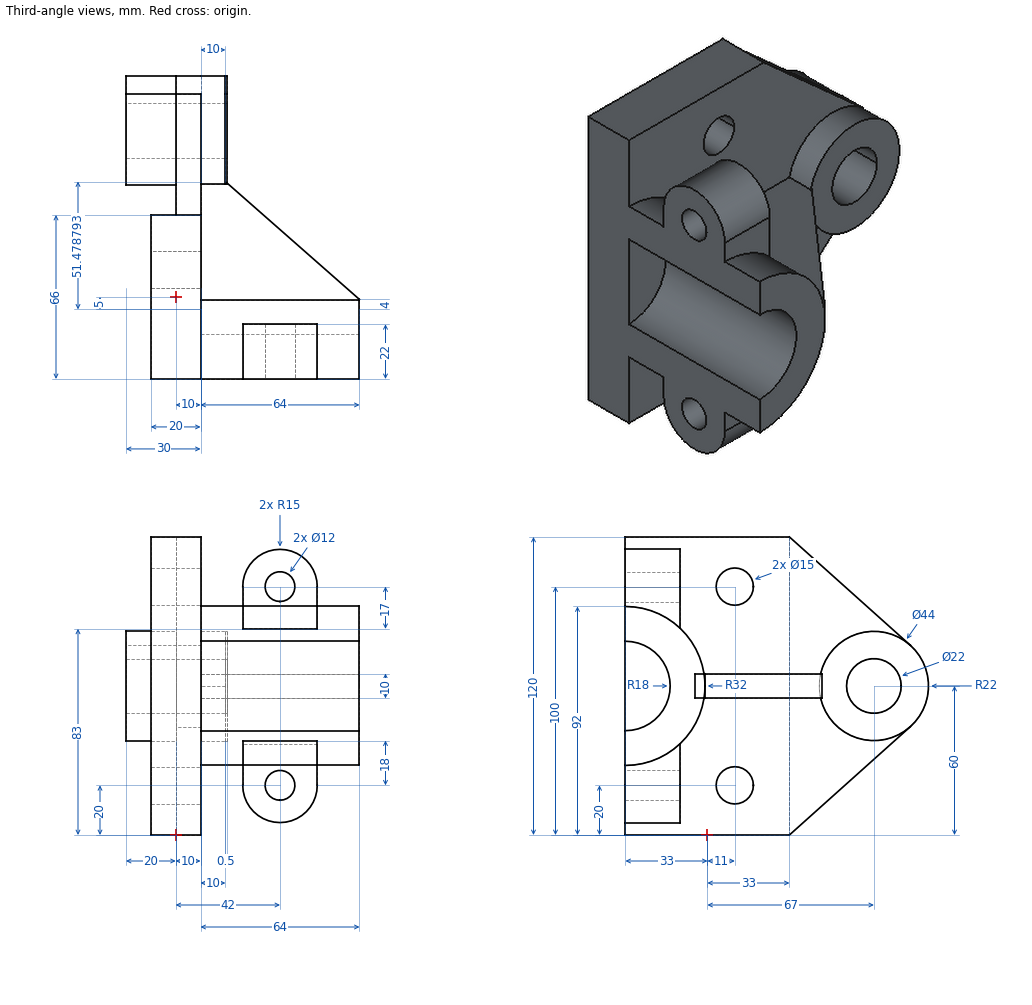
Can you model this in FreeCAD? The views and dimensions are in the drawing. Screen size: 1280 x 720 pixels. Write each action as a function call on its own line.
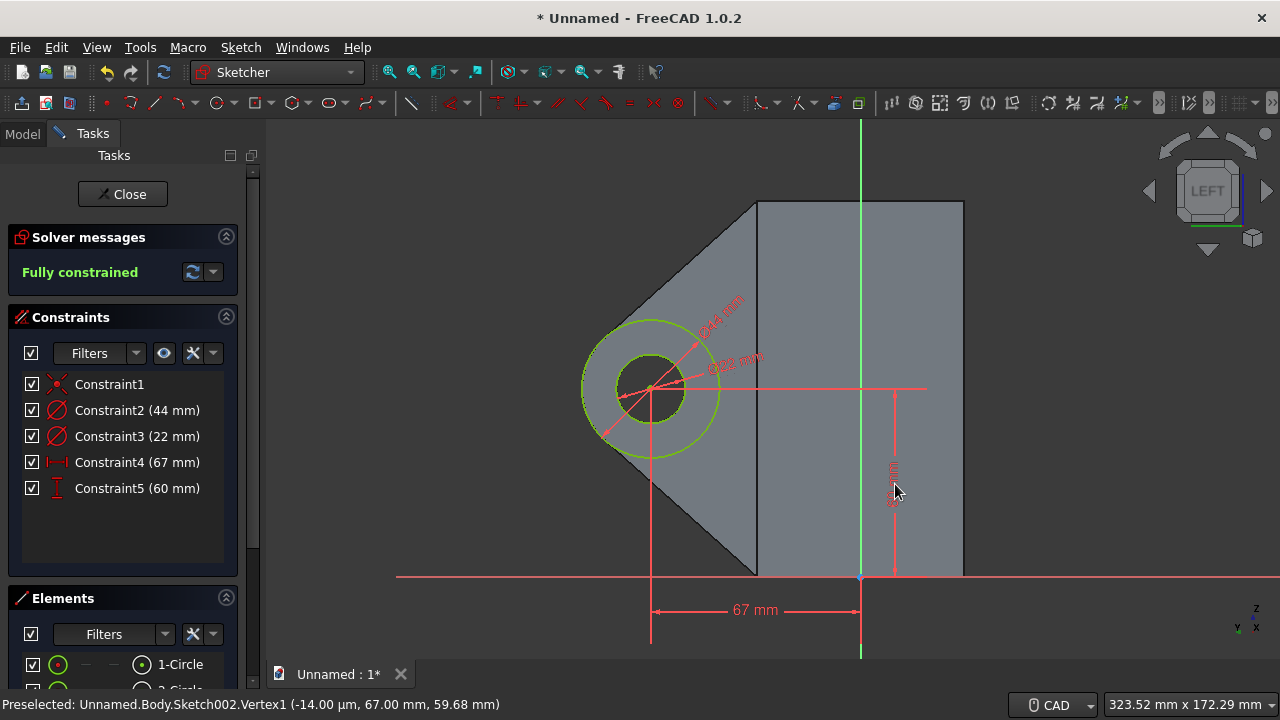
click(123, 194)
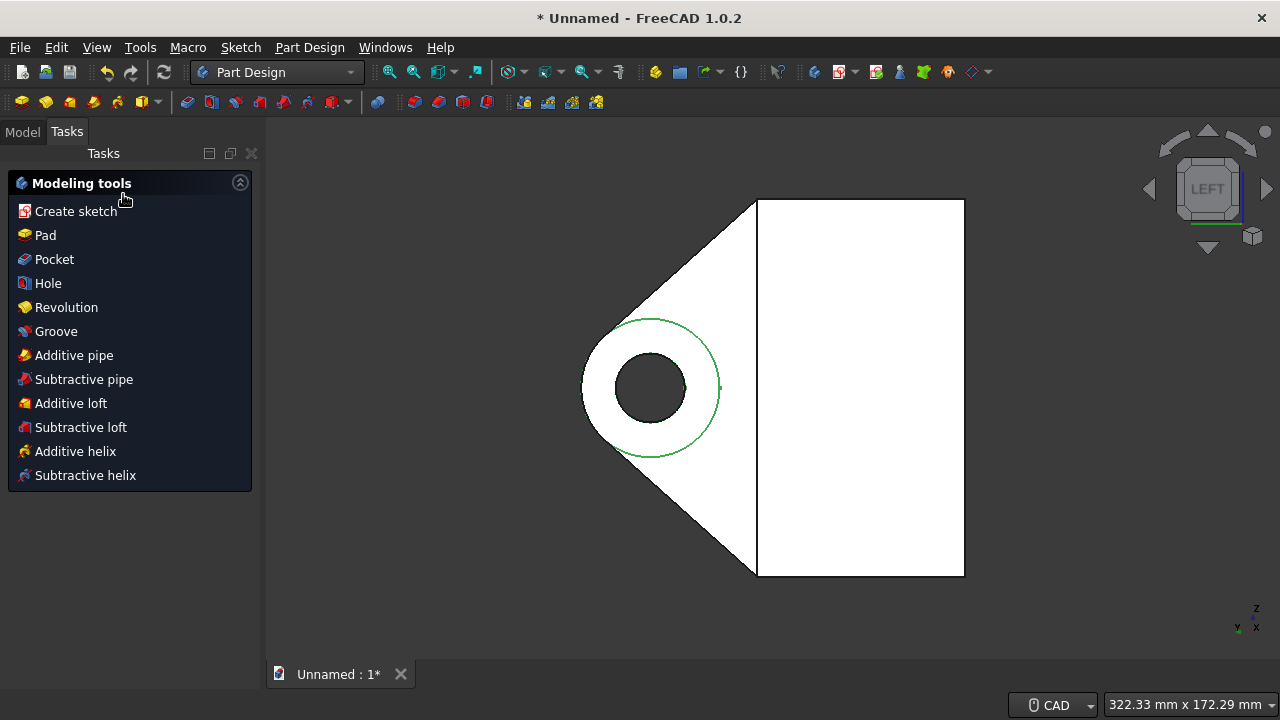
click(22, 102)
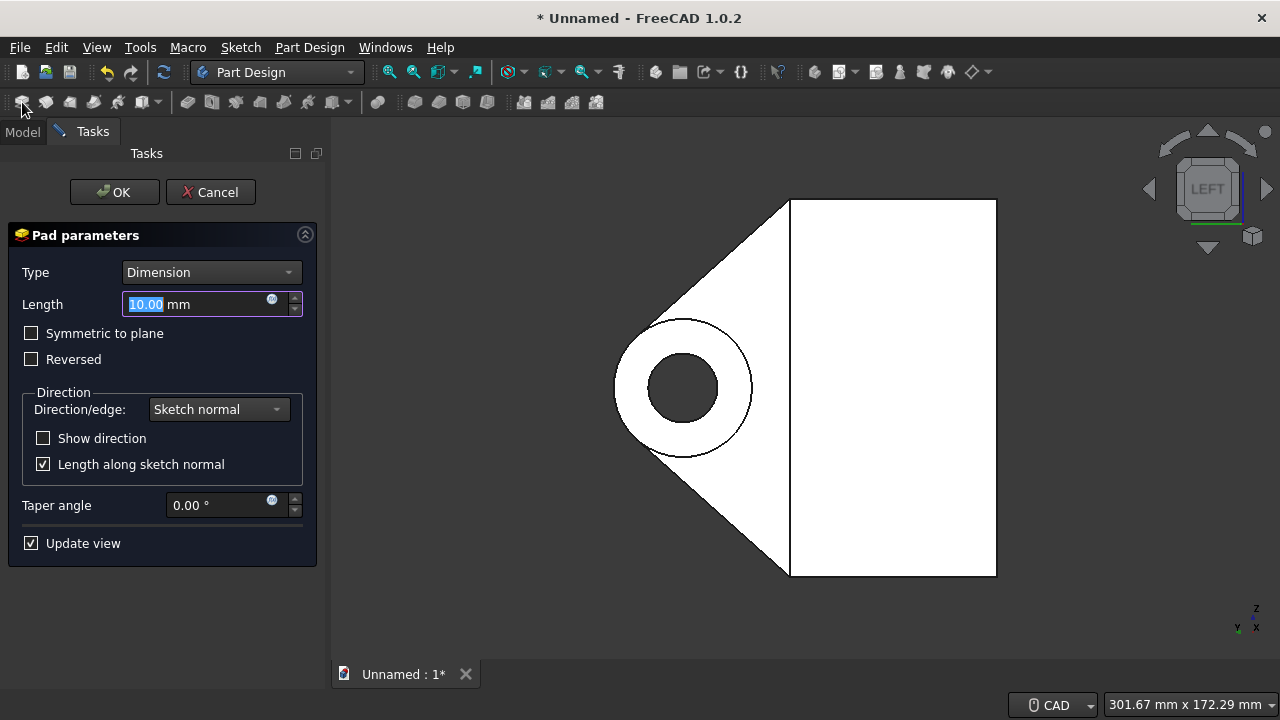
text(20)
key(Tab)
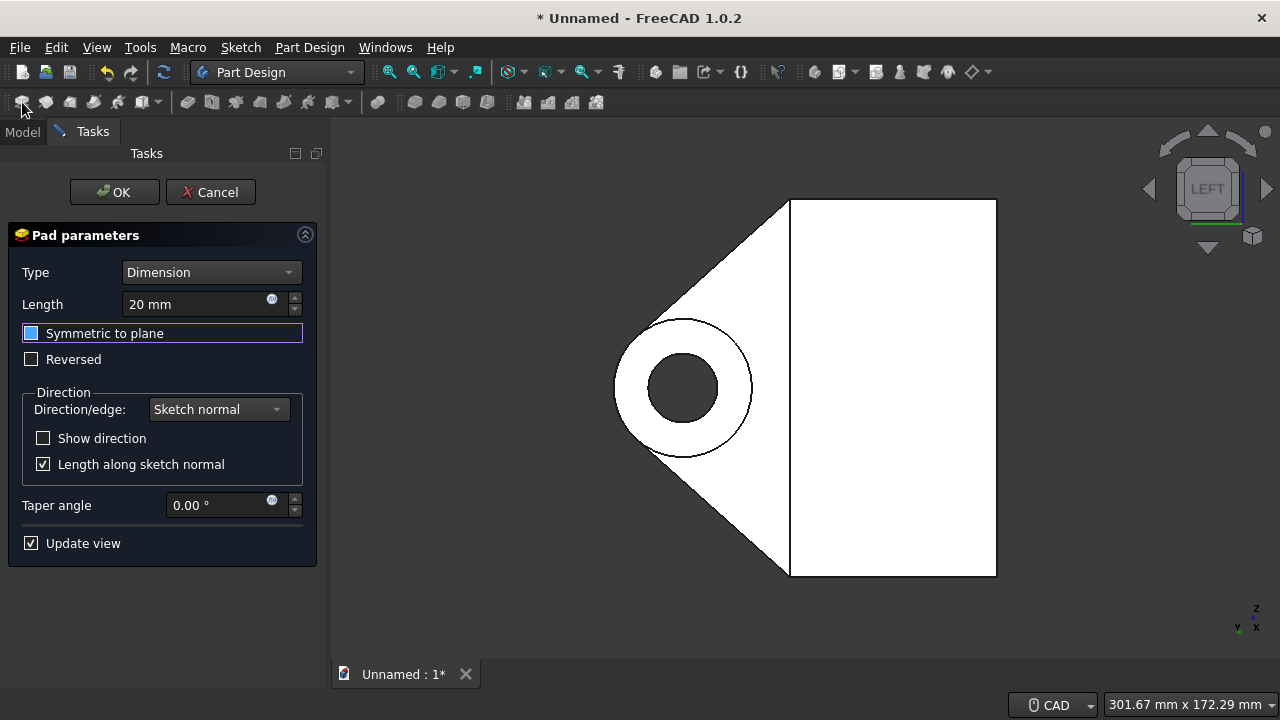
click(115, 192)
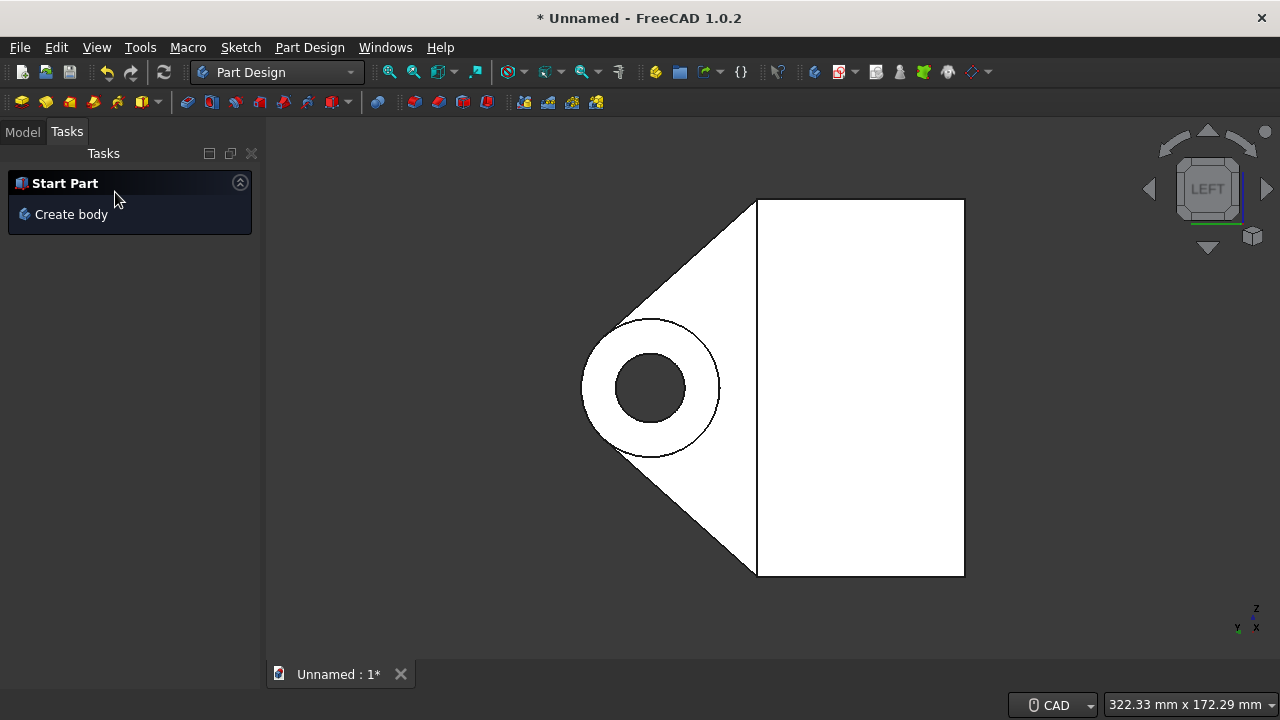
click(23, 131)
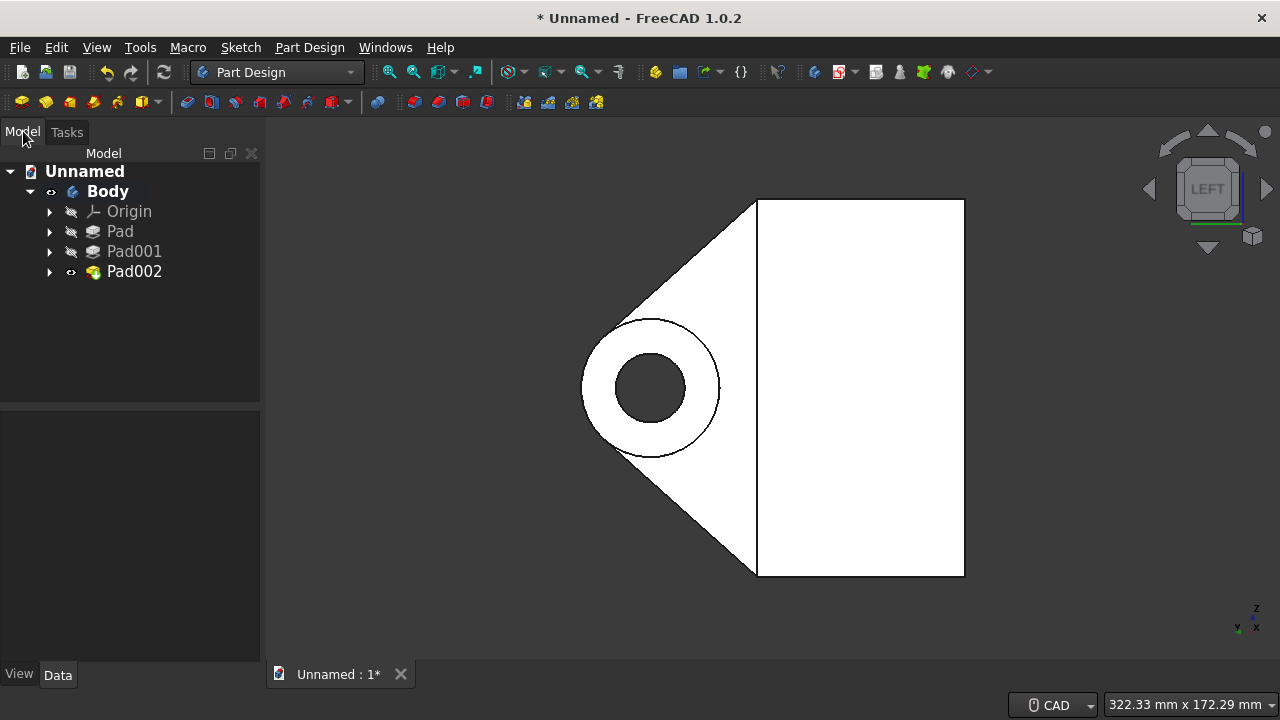
click(50, 212)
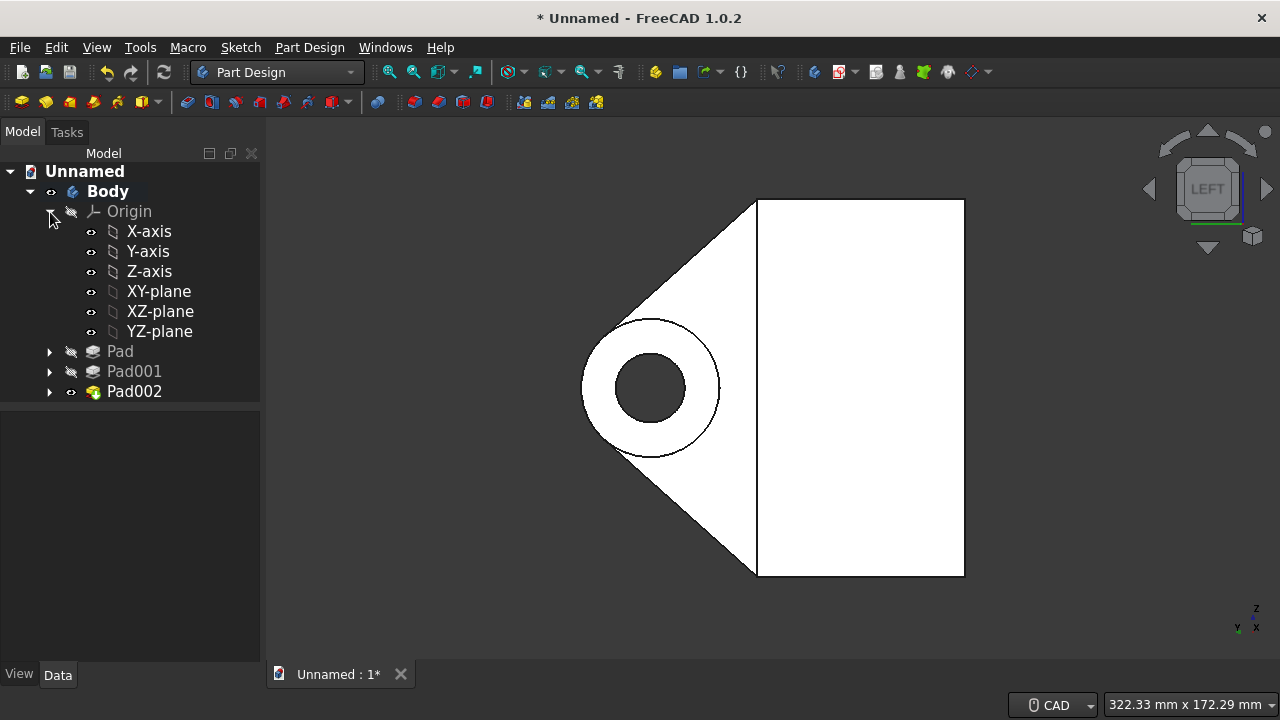
click(136, 332)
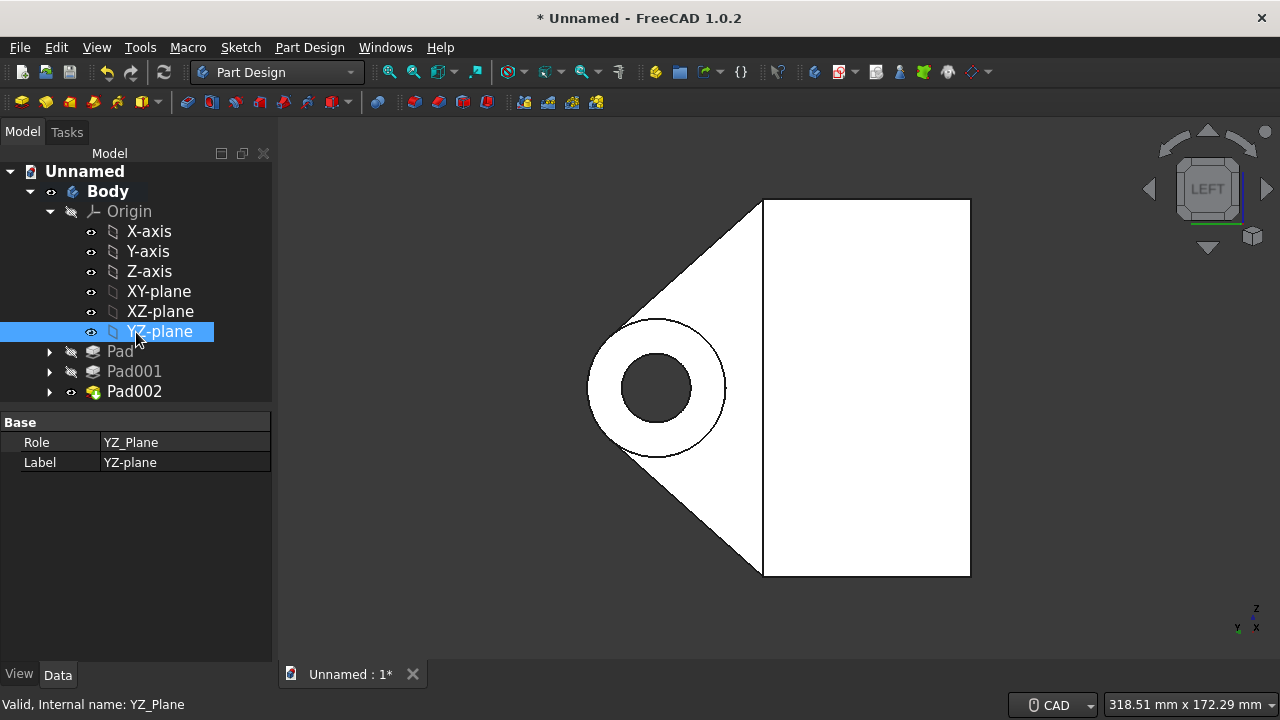
click(972, 72)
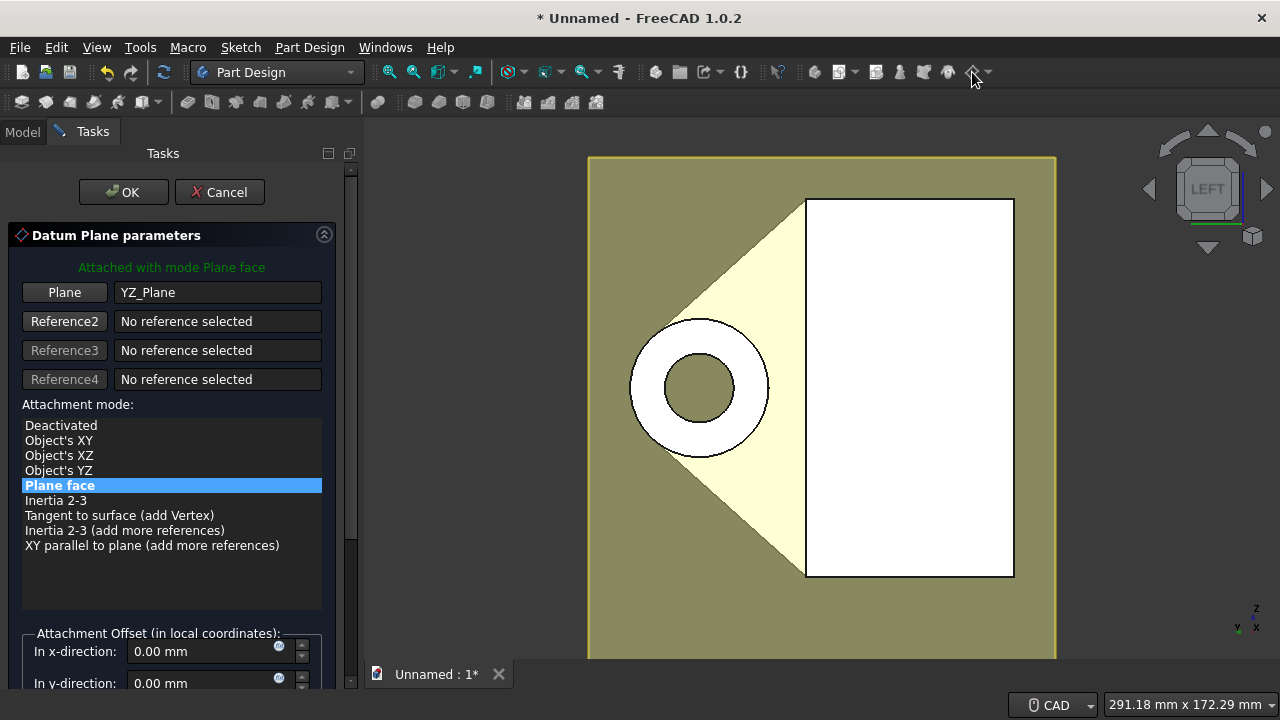
scroll(351, 426, down, 2)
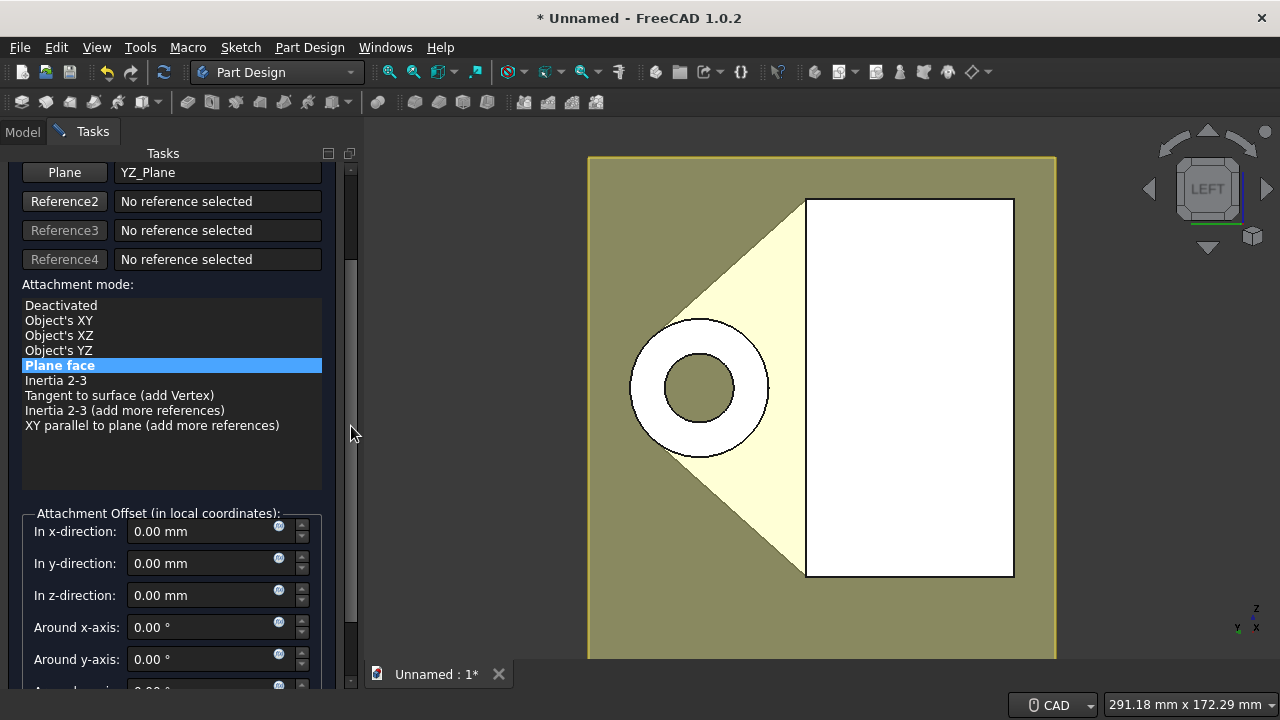
triple_click(210, 595)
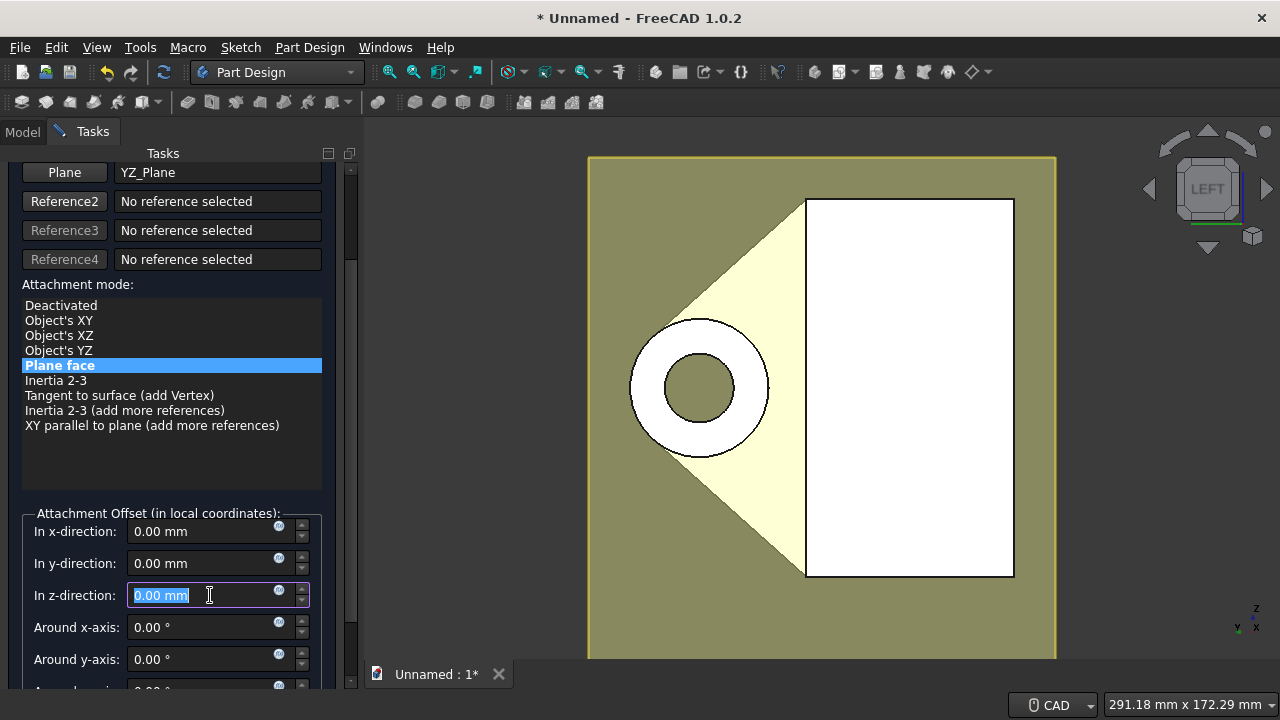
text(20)
key(Tab)